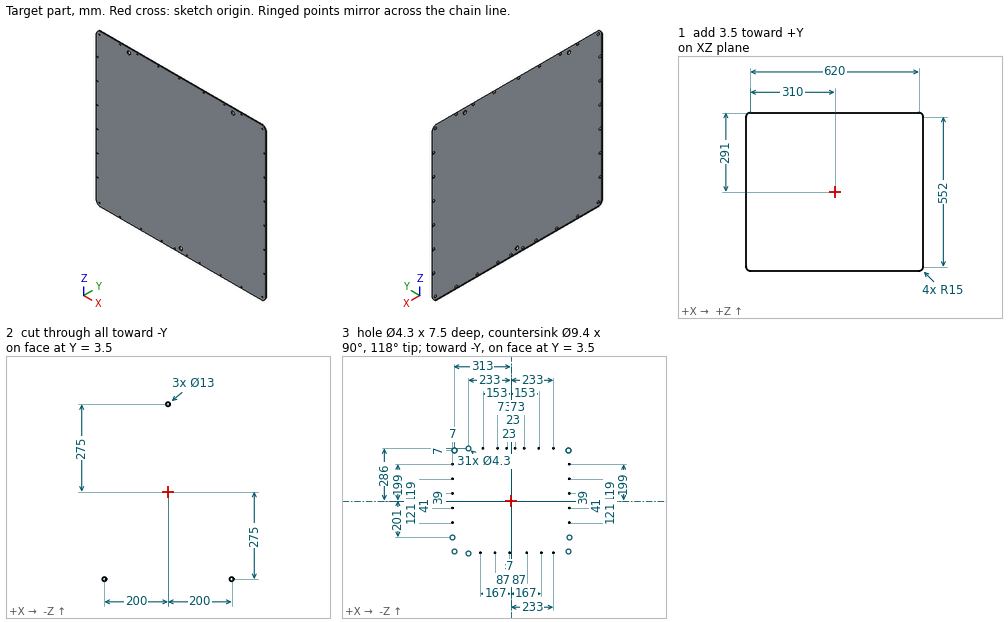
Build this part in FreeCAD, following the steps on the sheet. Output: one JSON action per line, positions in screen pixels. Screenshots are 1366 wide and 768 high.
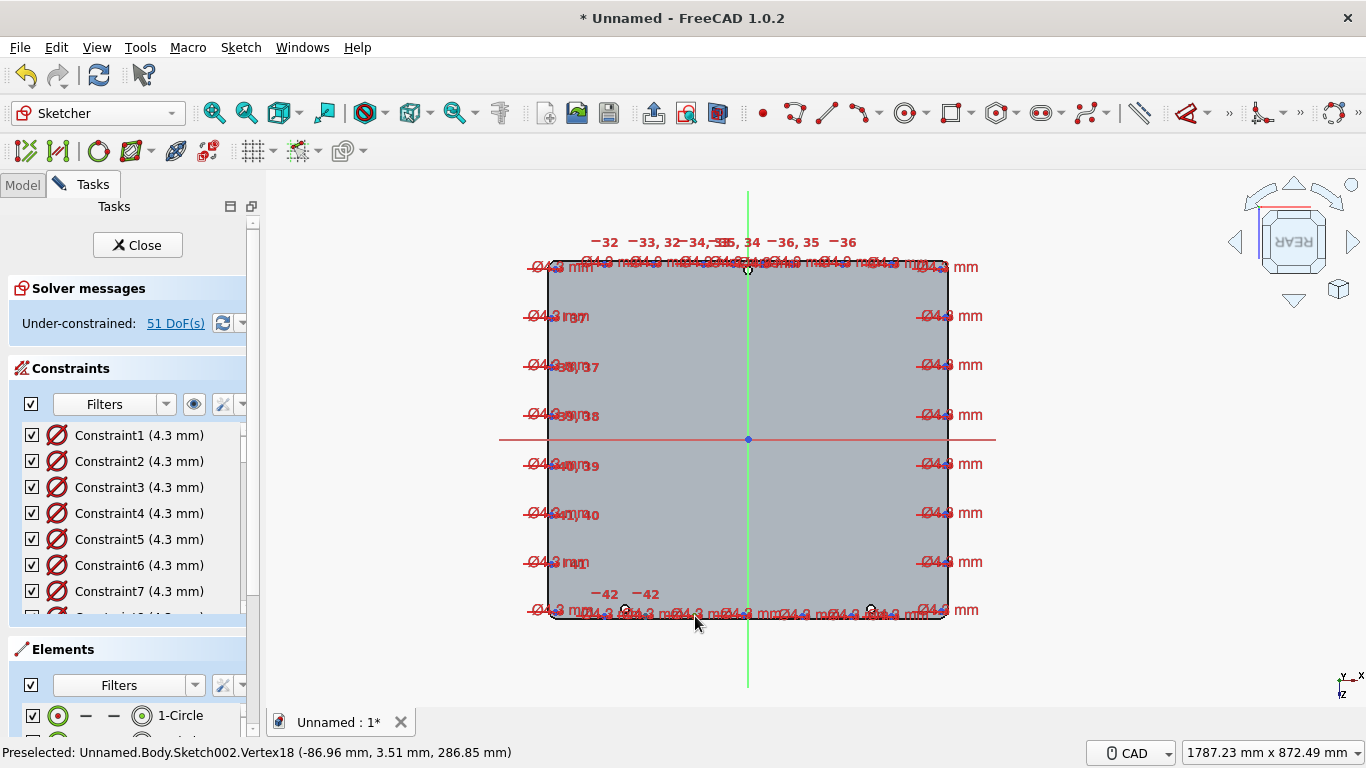
{"action": "key", "text": "h"}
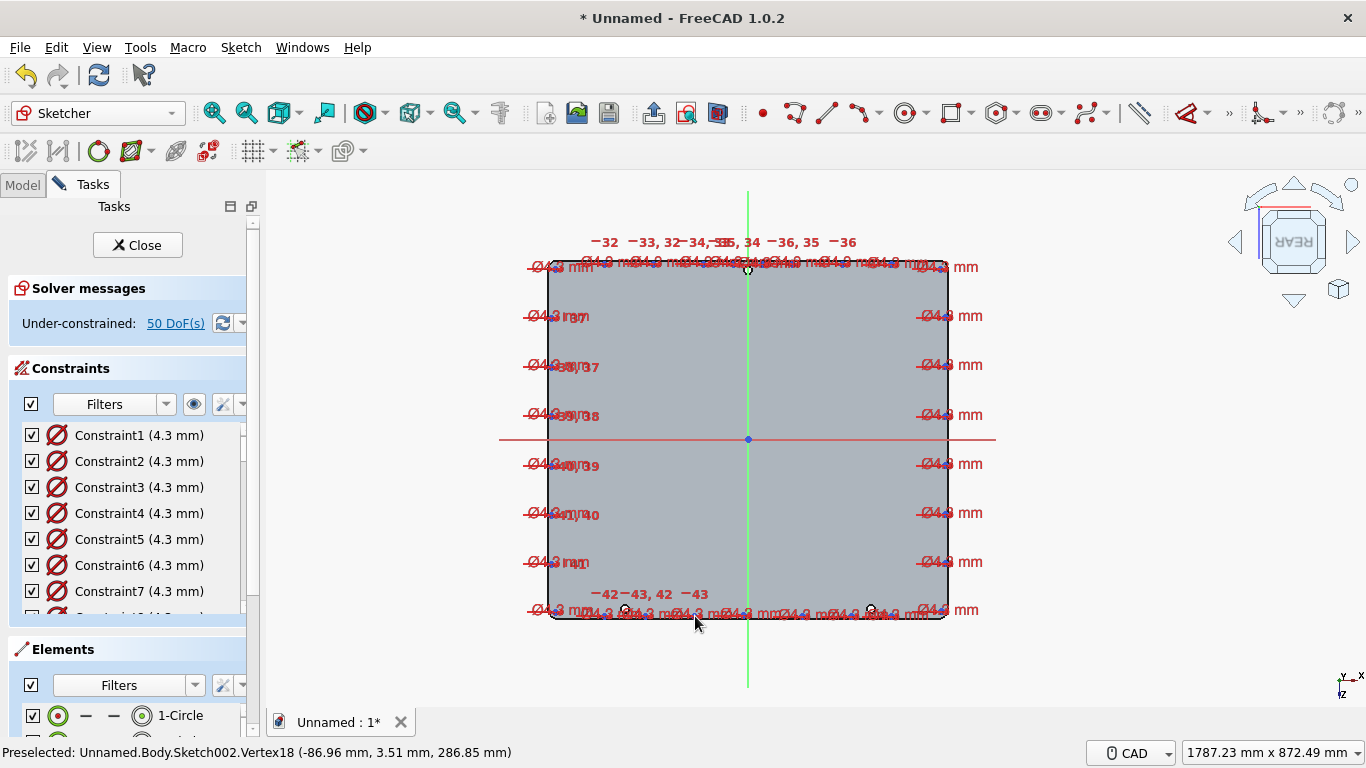
{"action": "left_click", "coordinate": [695, 616]}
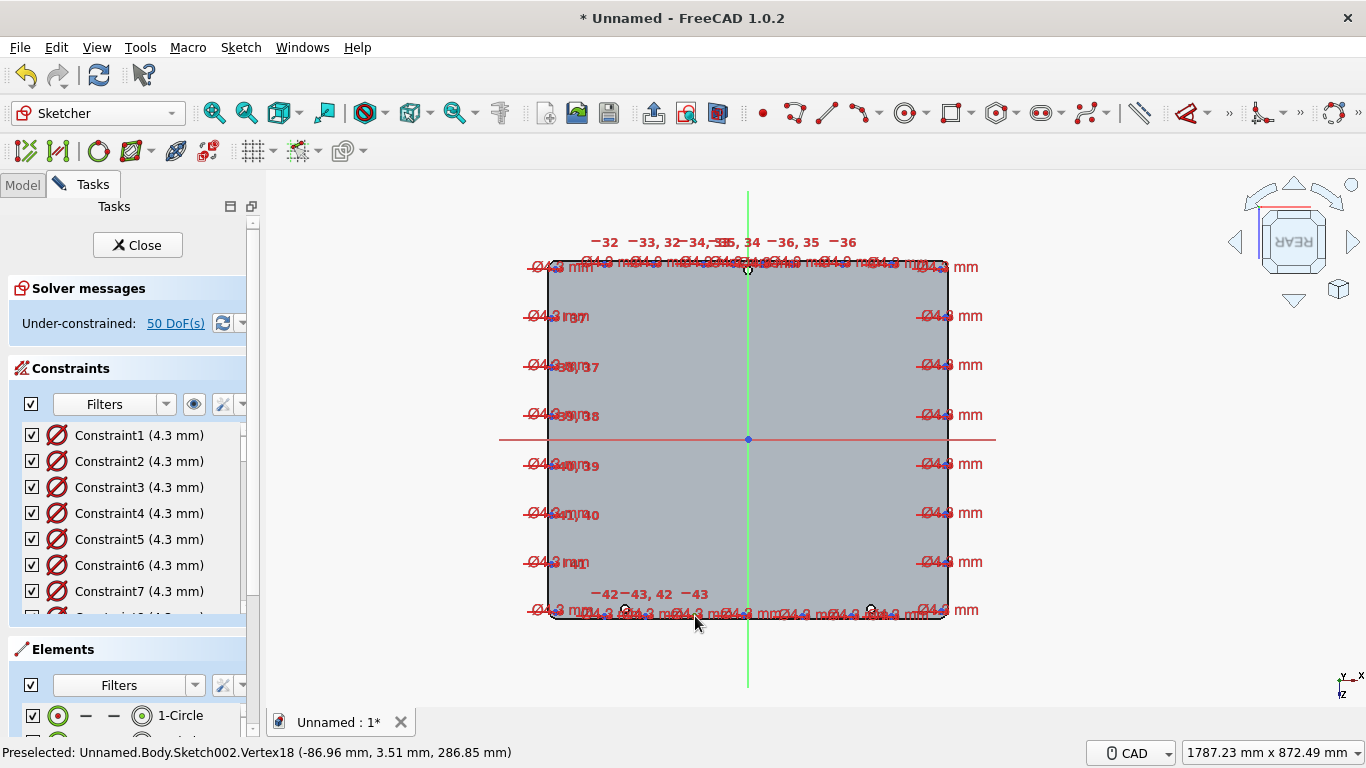
{"action": "left_click", "coordinate": [744, 616]}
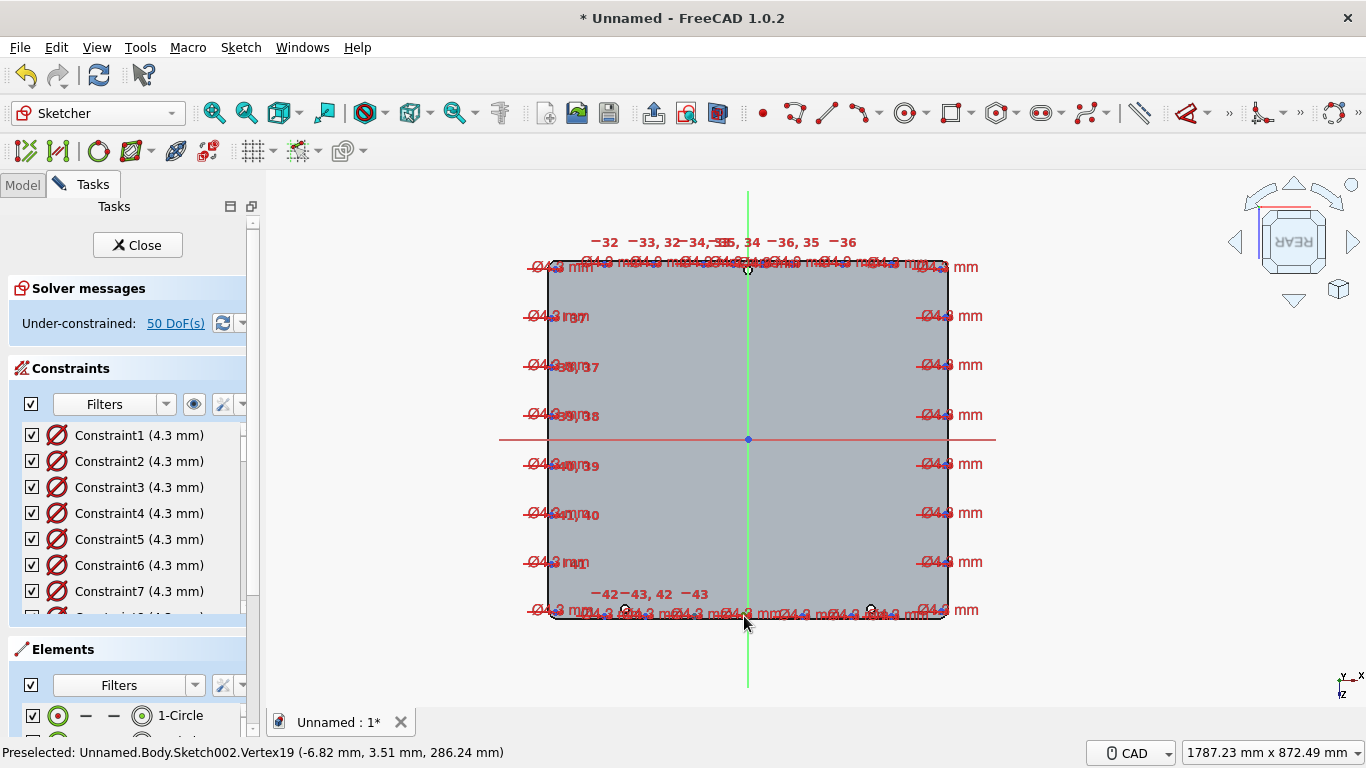
{"action": "key", "text": "h"}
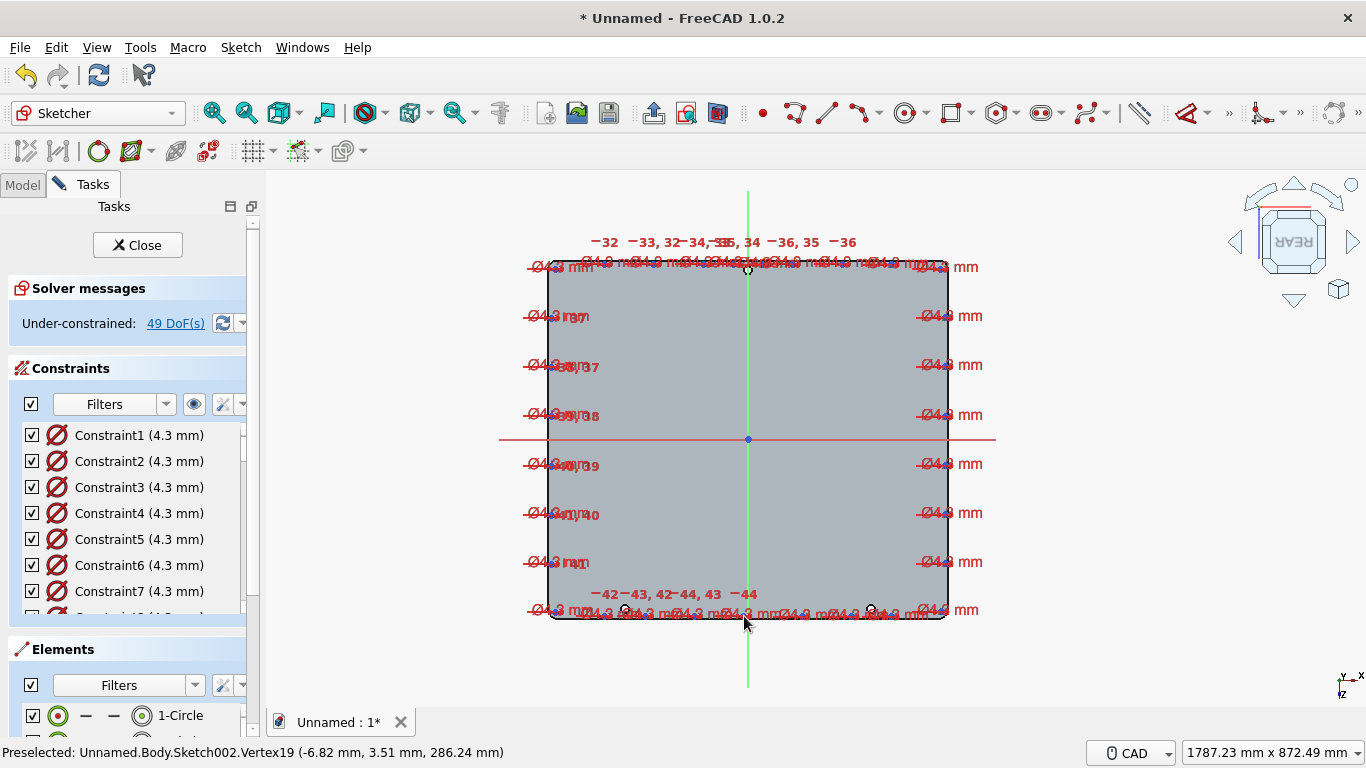
{"action": "left_click", "coordinate": [744, 616]}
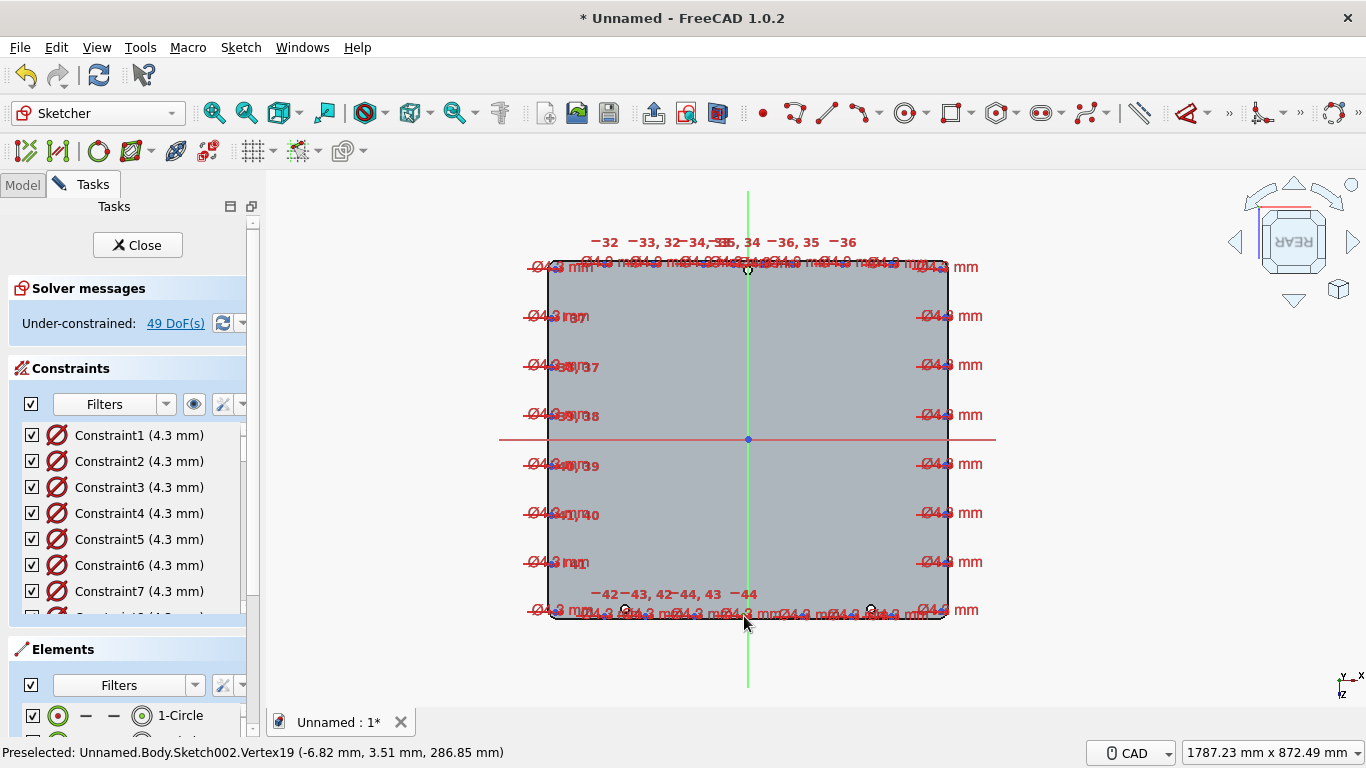
{"action": "left_click", "coordinate": [802, 617]}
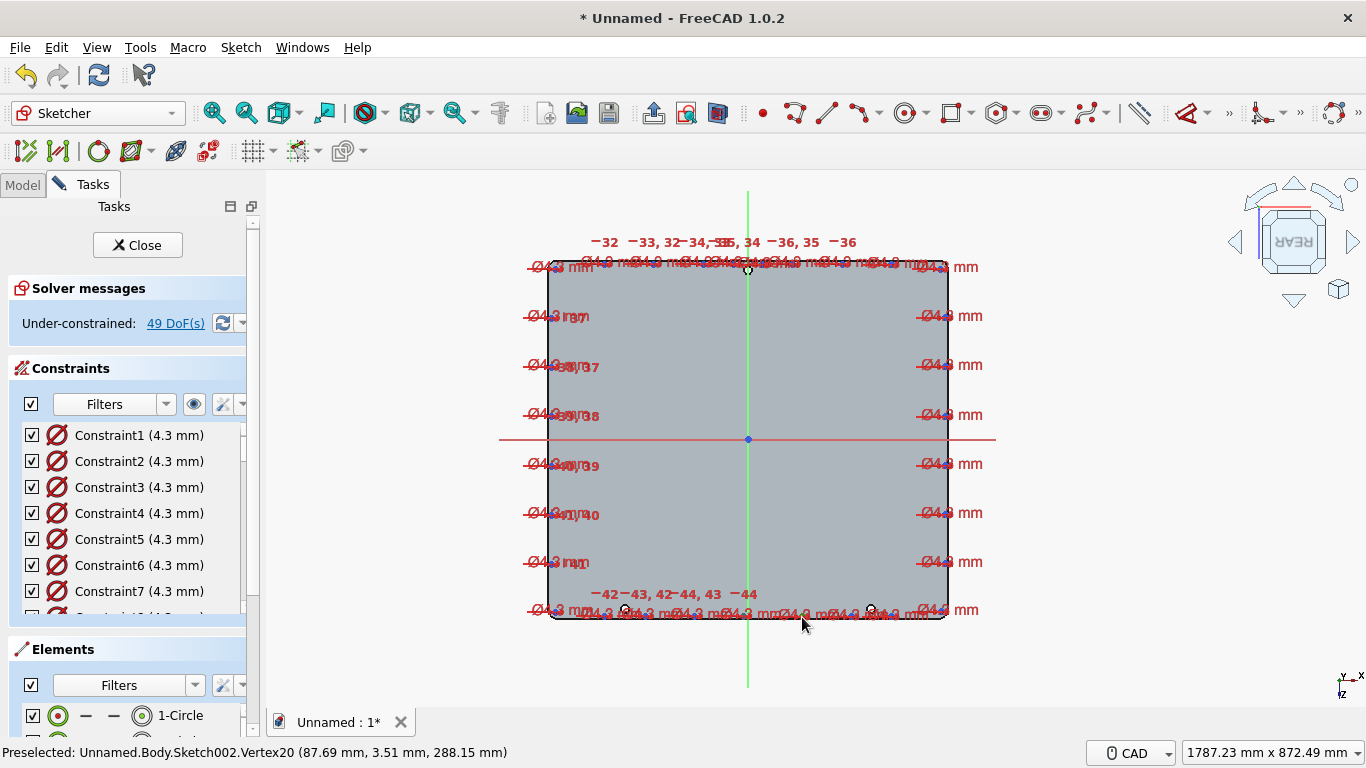
{"action": "key", "text": "h"}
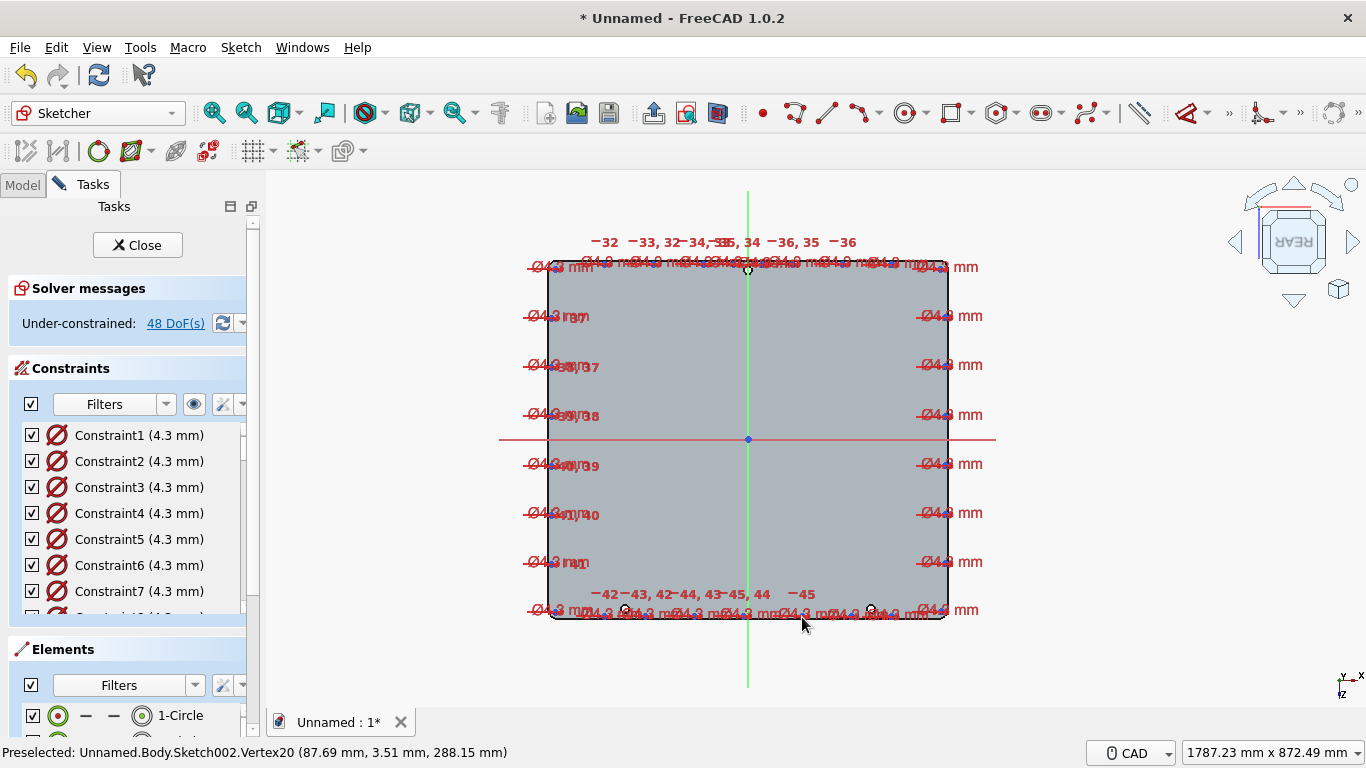
{"action": "left_click", "coordinate": [802, 616]}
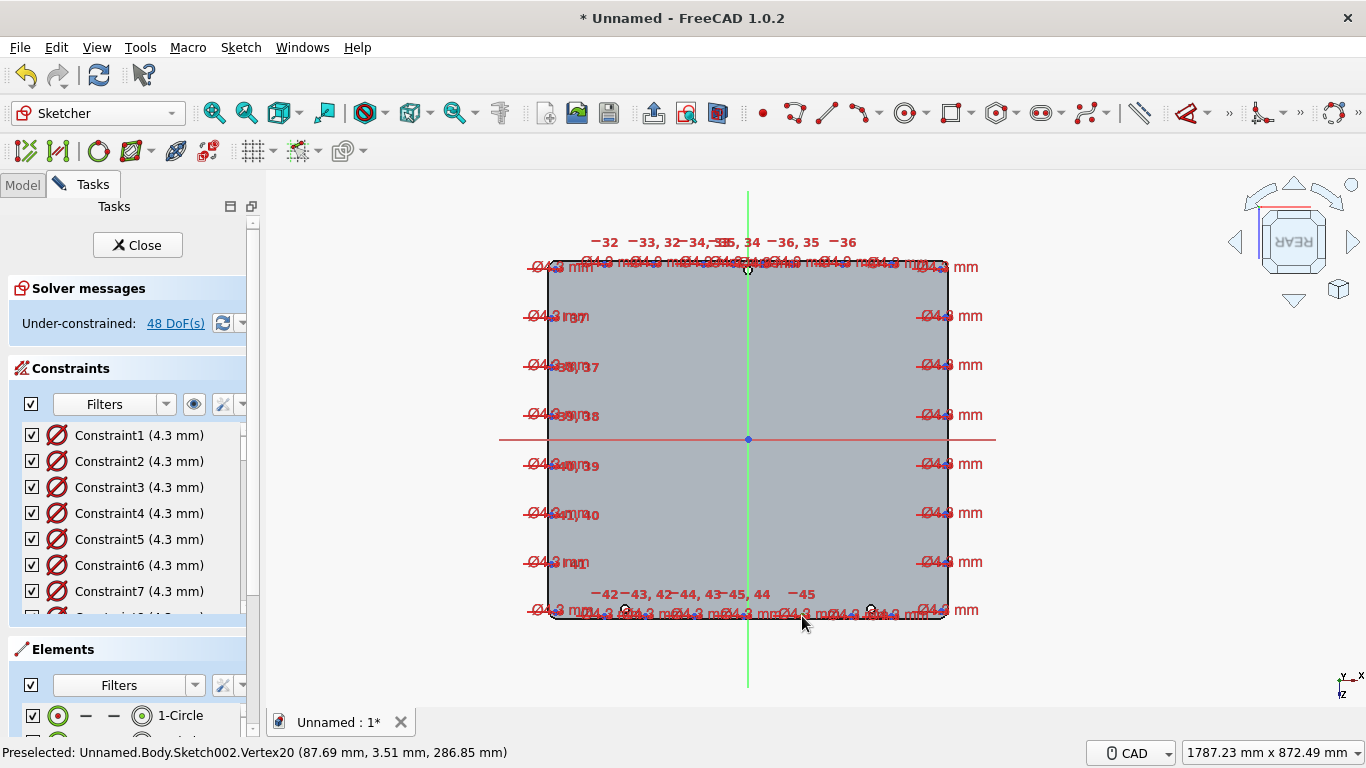
{"action": "left_click", "coordinate": [851, 617]}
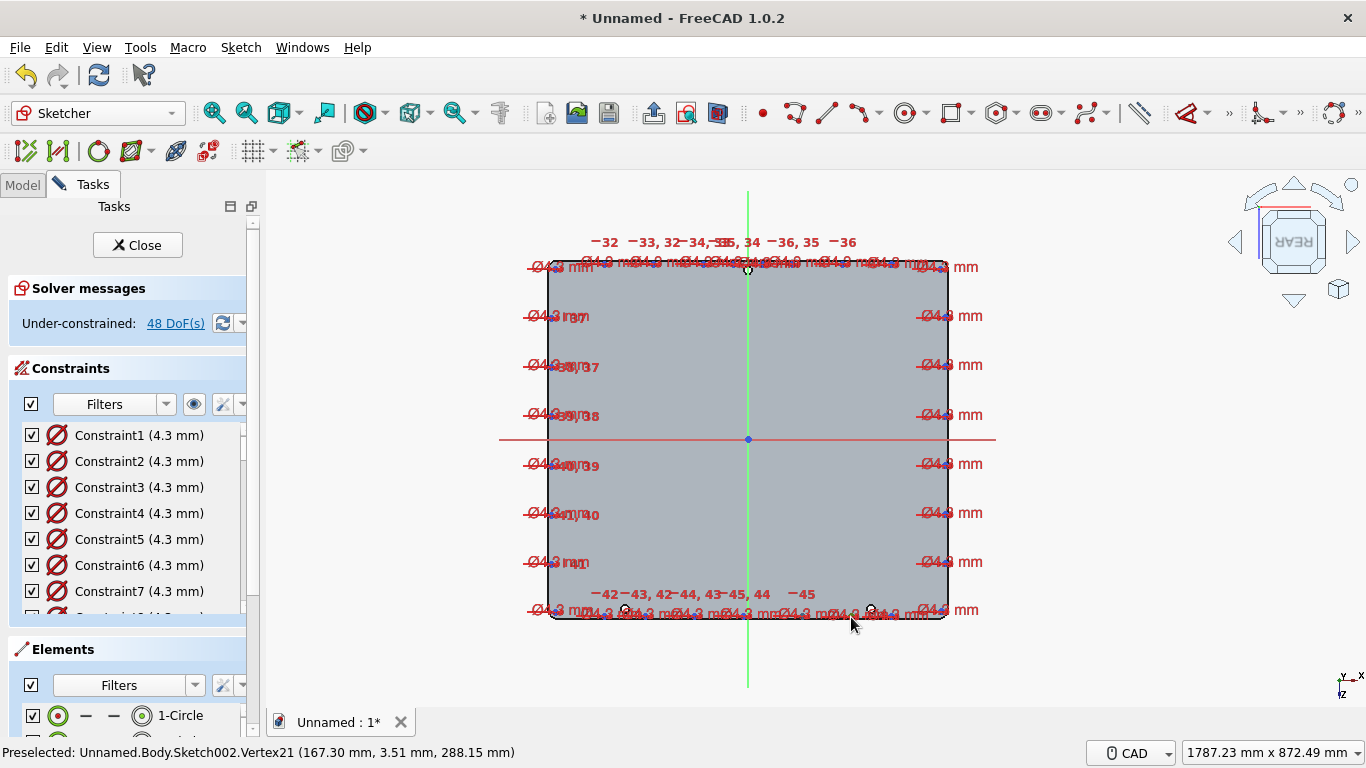
{"action": "key", "text": "h"}